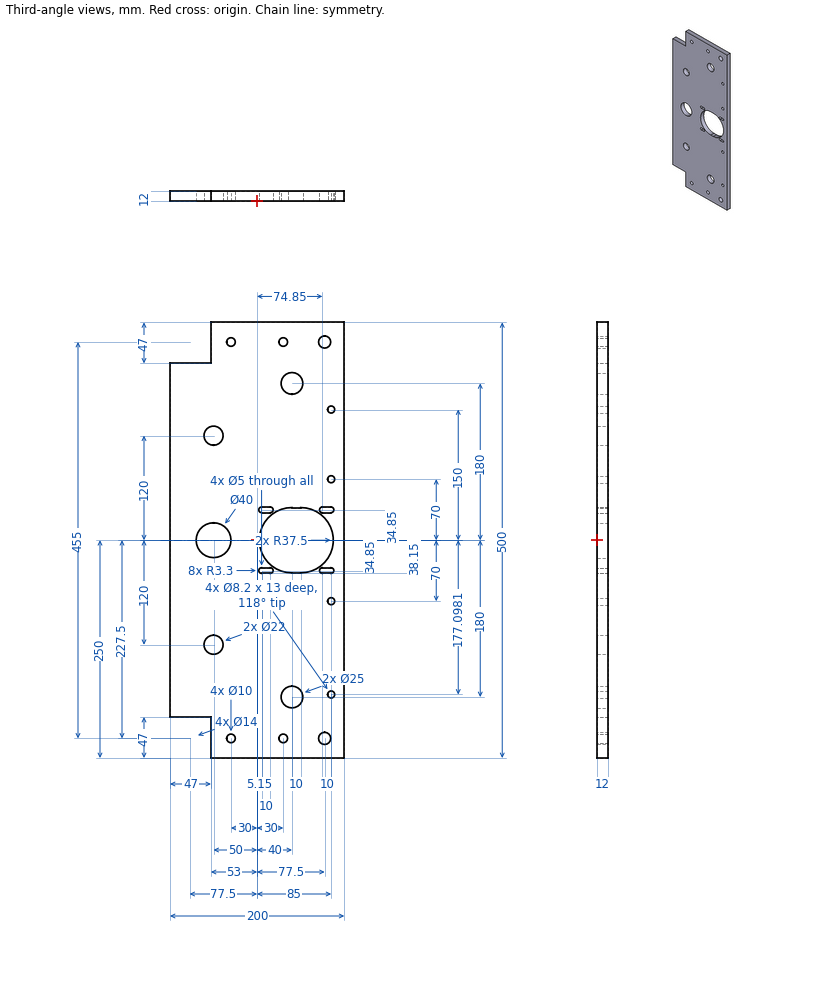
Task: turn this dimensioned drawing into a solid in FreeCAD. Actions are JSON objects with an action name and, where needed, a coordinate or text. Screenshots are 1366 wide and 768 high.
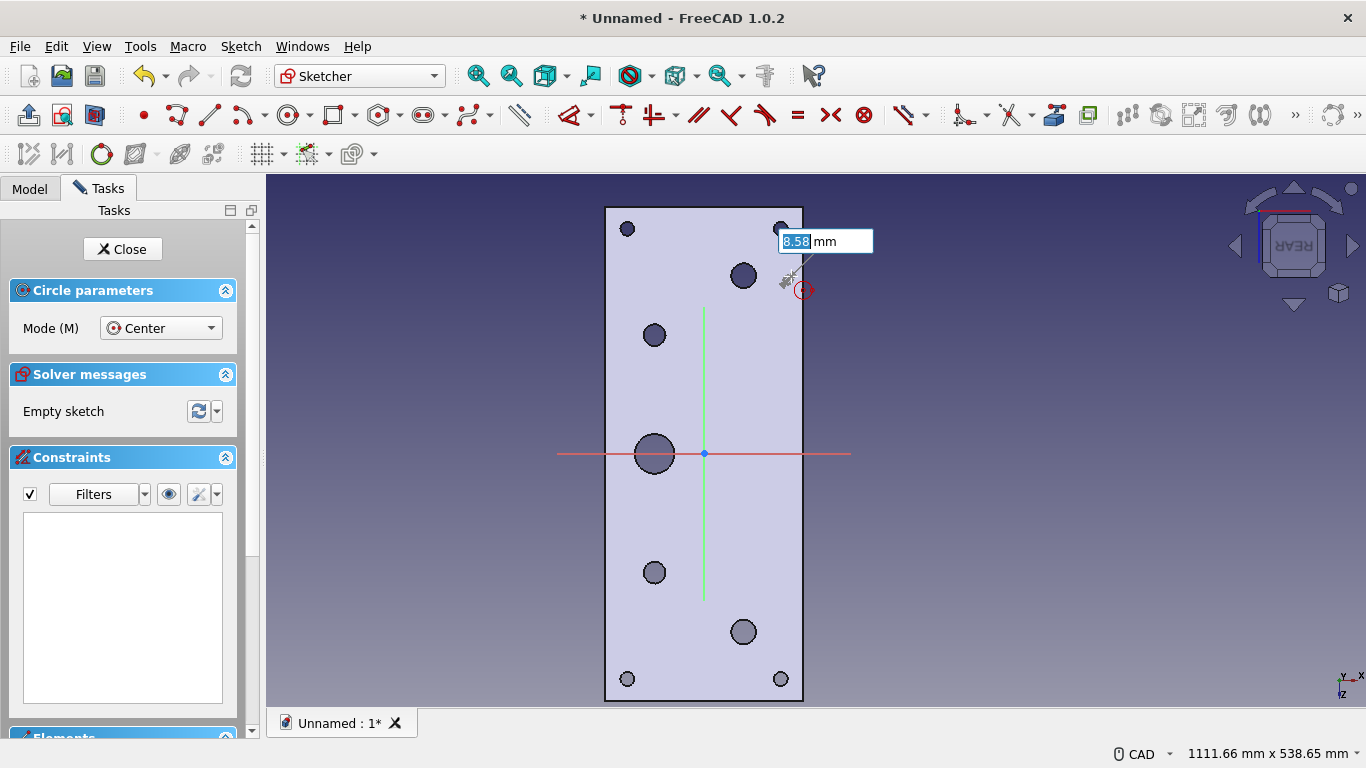
{"action": "type", "text": "8.2"}
{"action": "key", "text": "Return"}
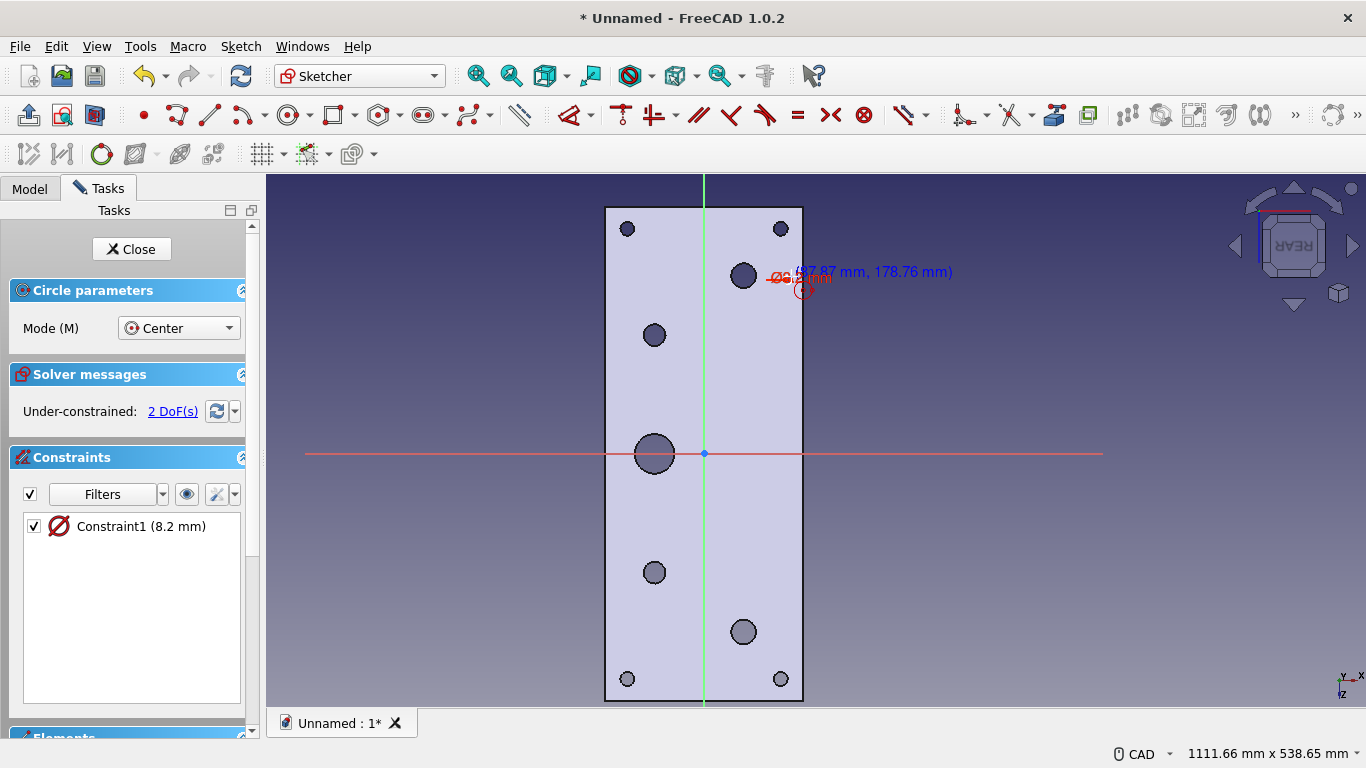
{"action": "scroll", "coordinate": [788, 385], "scroll_direction": "up", "scroll_amount": 9}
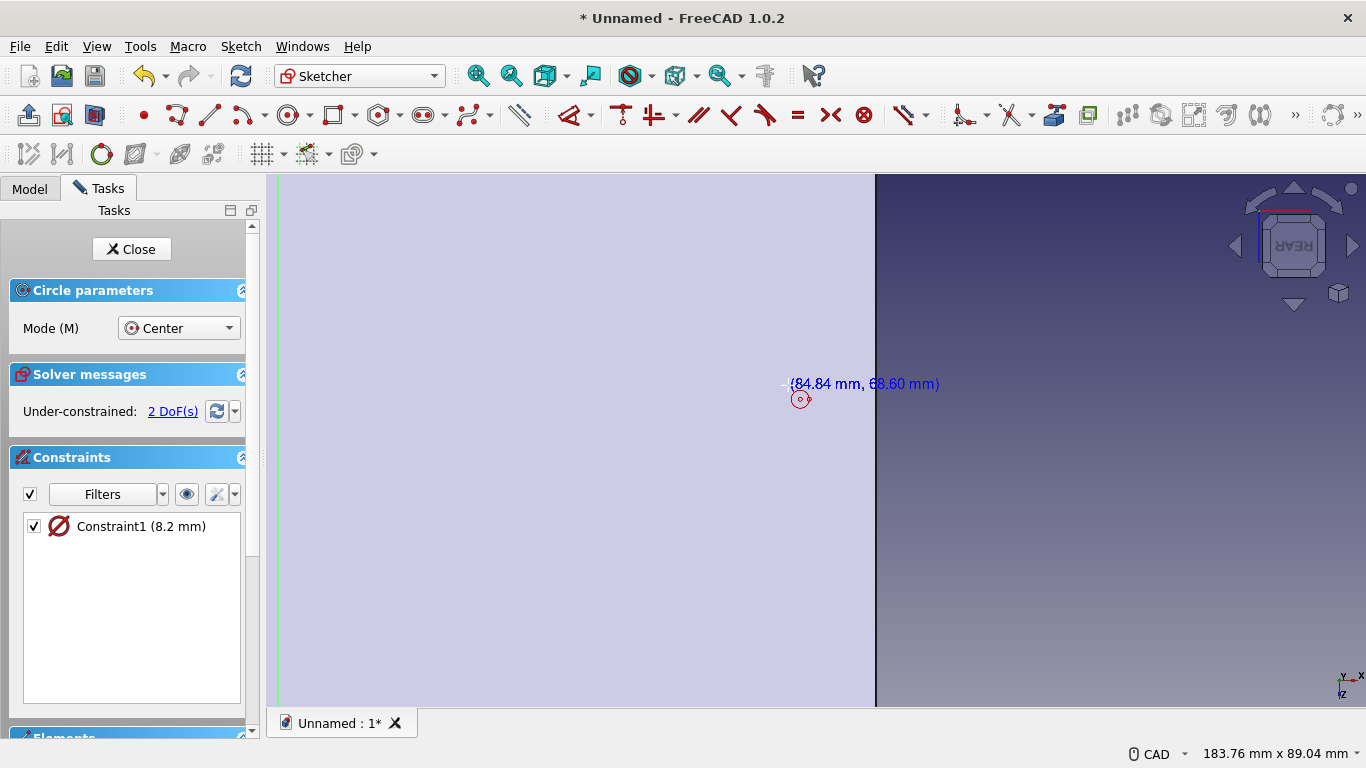
{"action": "scroll", "coordinate": [788, 385], "scroll_direction": "down", "scroll_amount": 9}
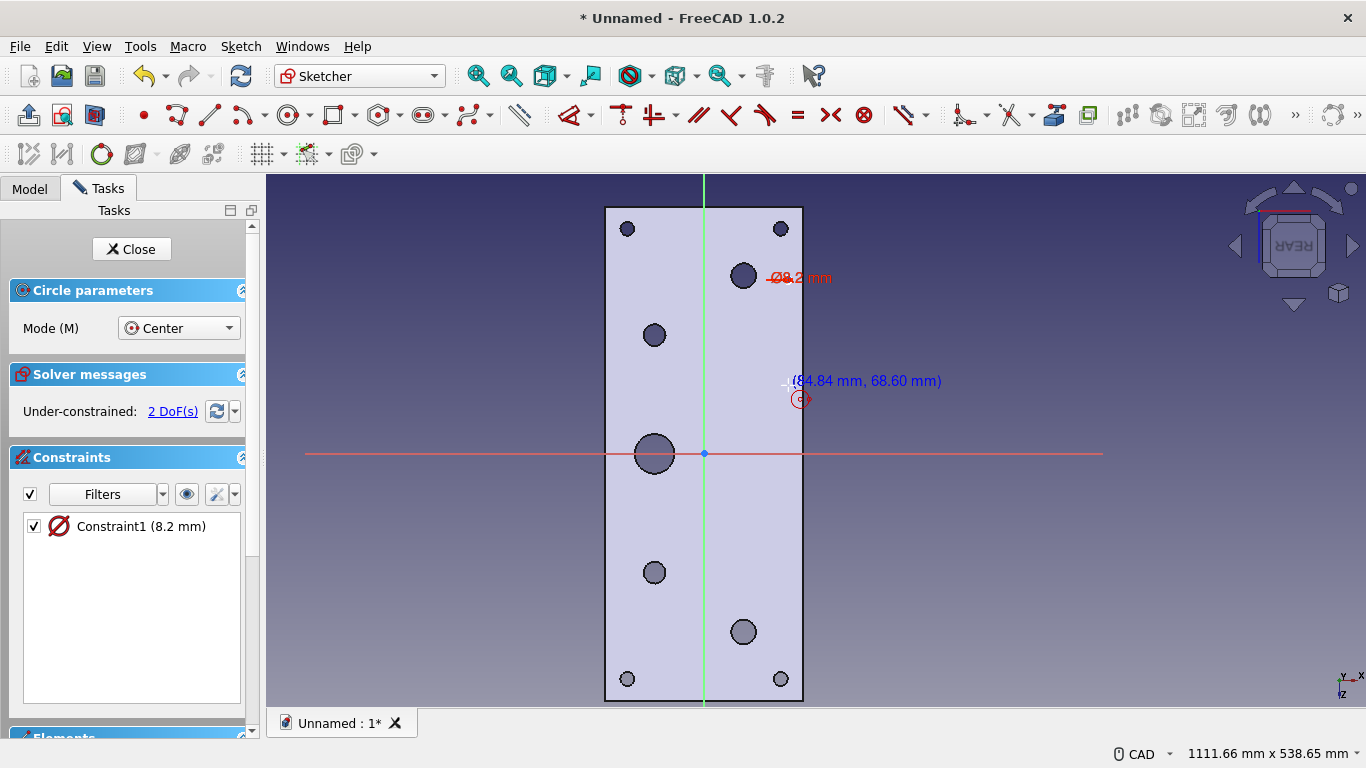
{"action": "left_click", "coordinate": [788, 385]}
{"action": "mouse_move", "coordinate": [791, 382]}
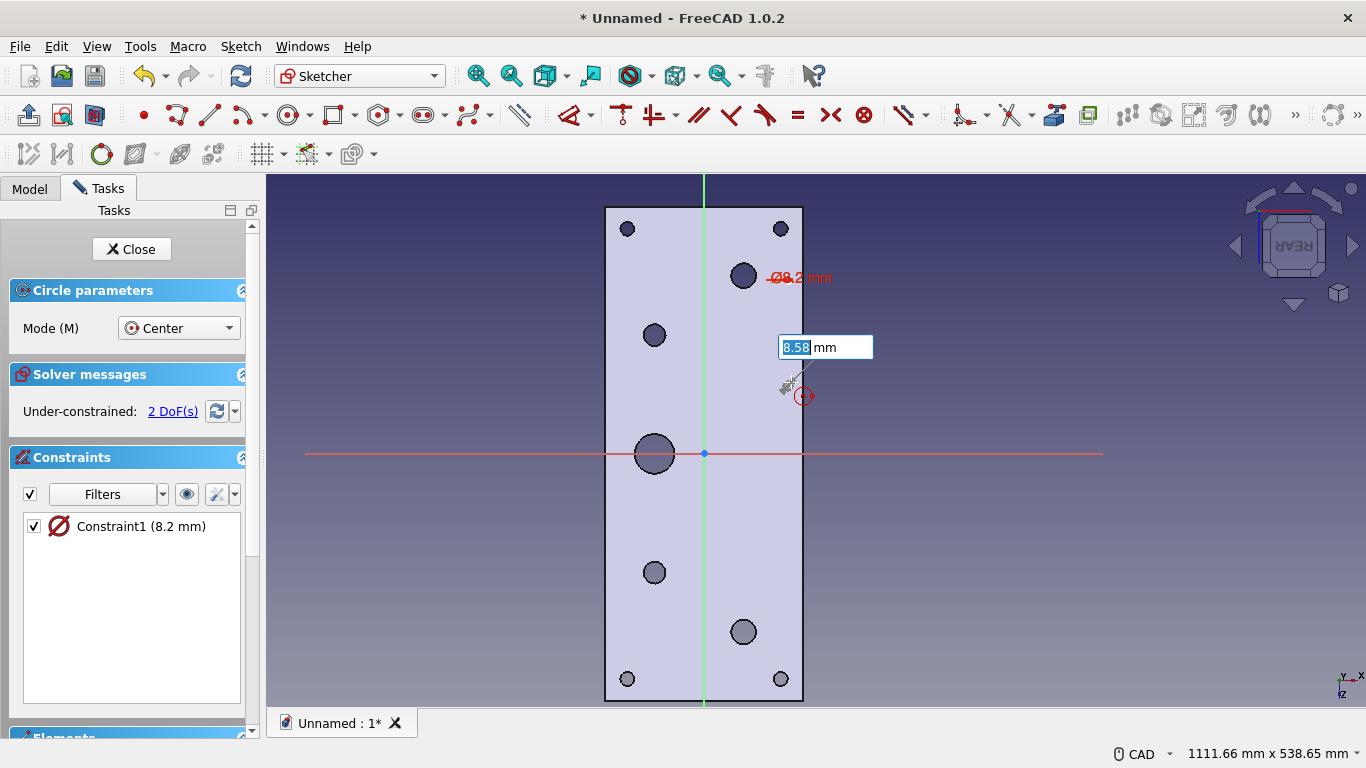
{"action": "type", "text": "8.2"}
{"action": "key", "text": "Return"}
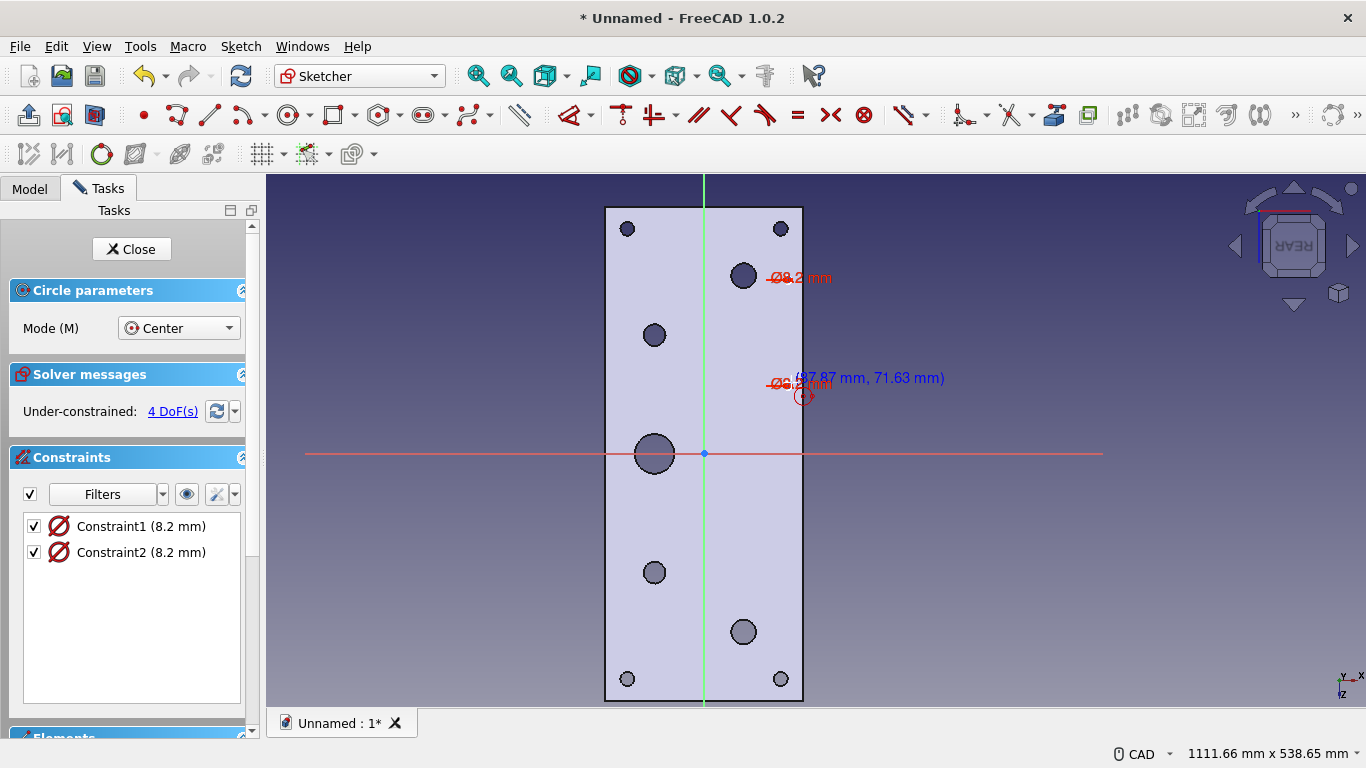
{"action": "scroll", "coordinate": [788, 523], "scroll_direction": "up", "scroll_amount": 9}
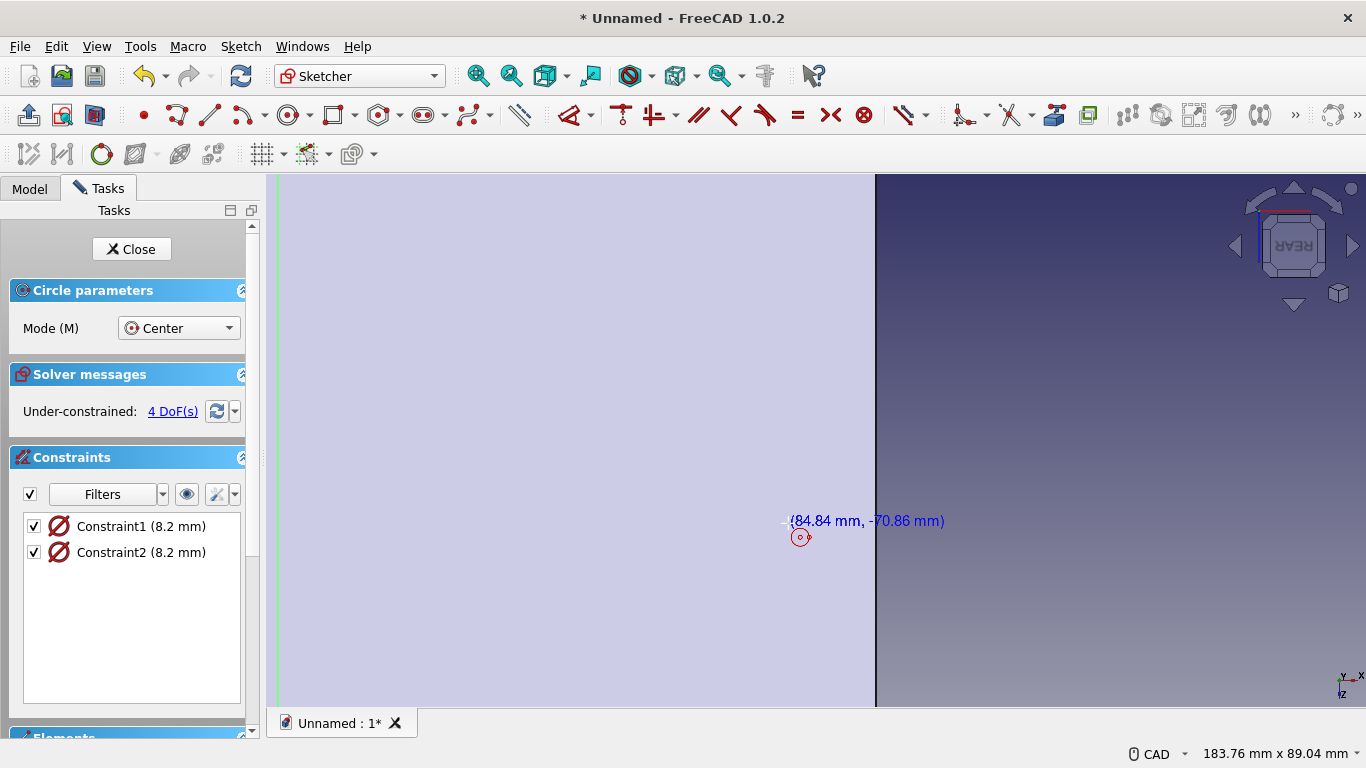
{"action": "scroll", "coordinate": [788, 524], "scroll_direction": "down", "scroll_amount": 9}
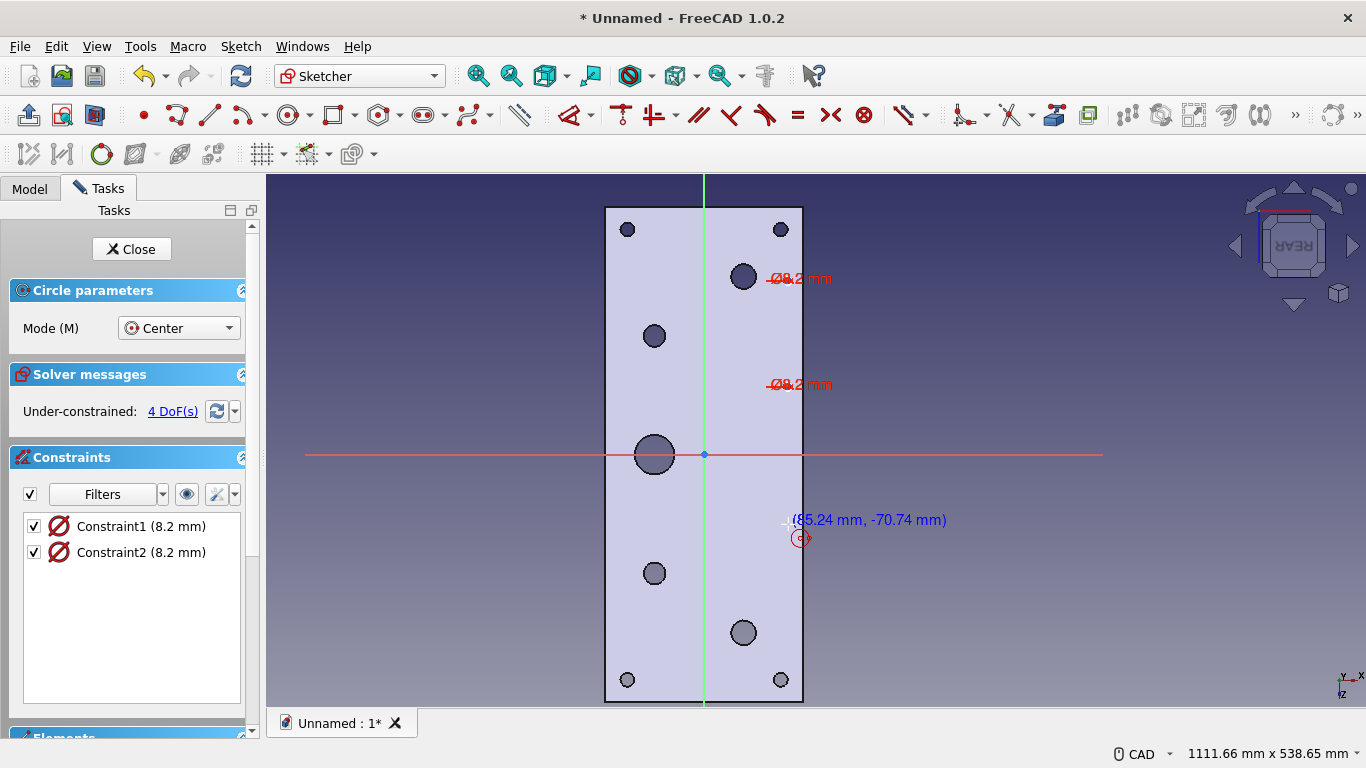
{"action": "left_click", "coordinate": [788, 524]}
{"action": "mouse_move", "coordinate": [791, 521]}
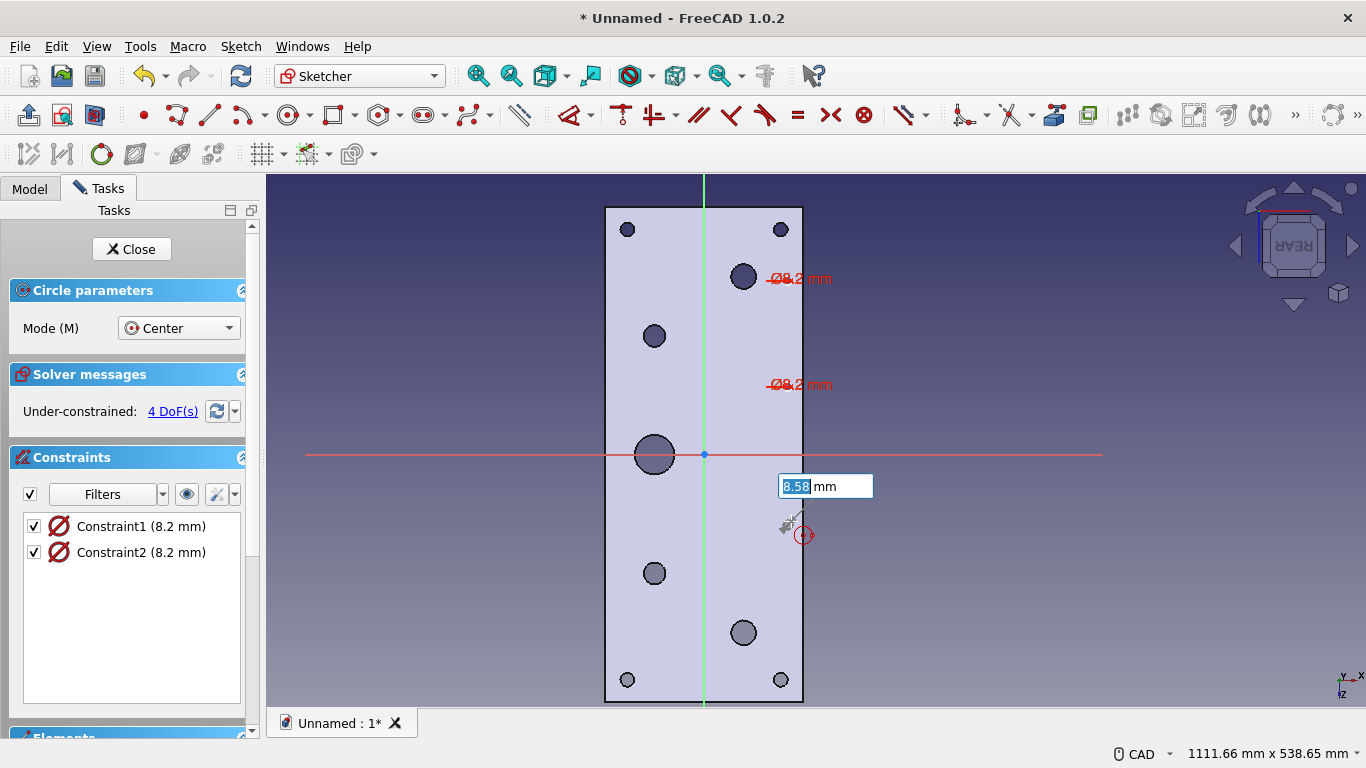
{"action": "type", "text": "8.2"}
{"action": "key", "text": "Return"}